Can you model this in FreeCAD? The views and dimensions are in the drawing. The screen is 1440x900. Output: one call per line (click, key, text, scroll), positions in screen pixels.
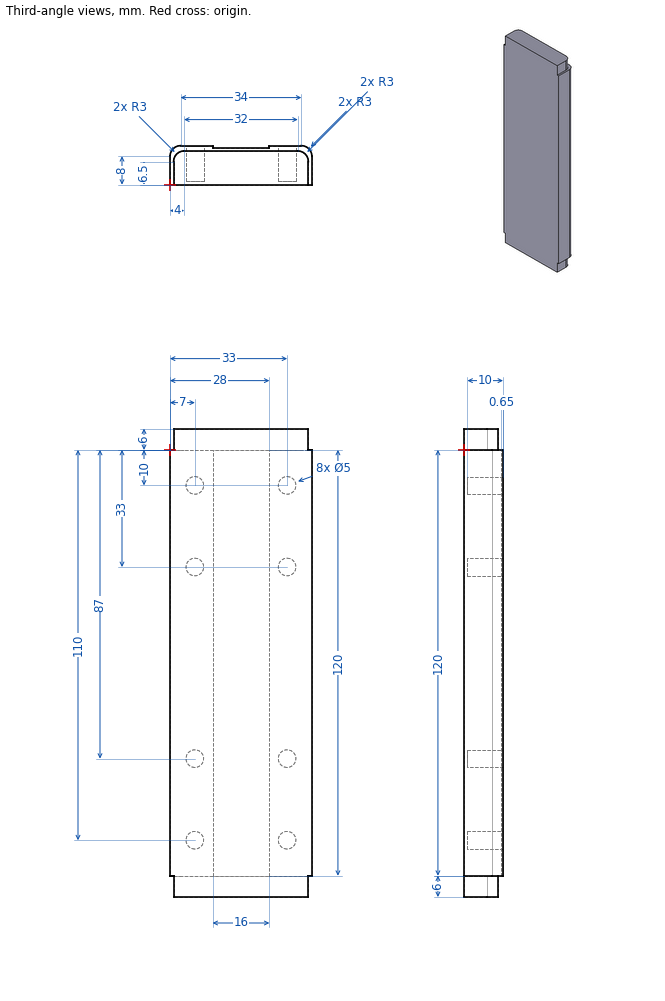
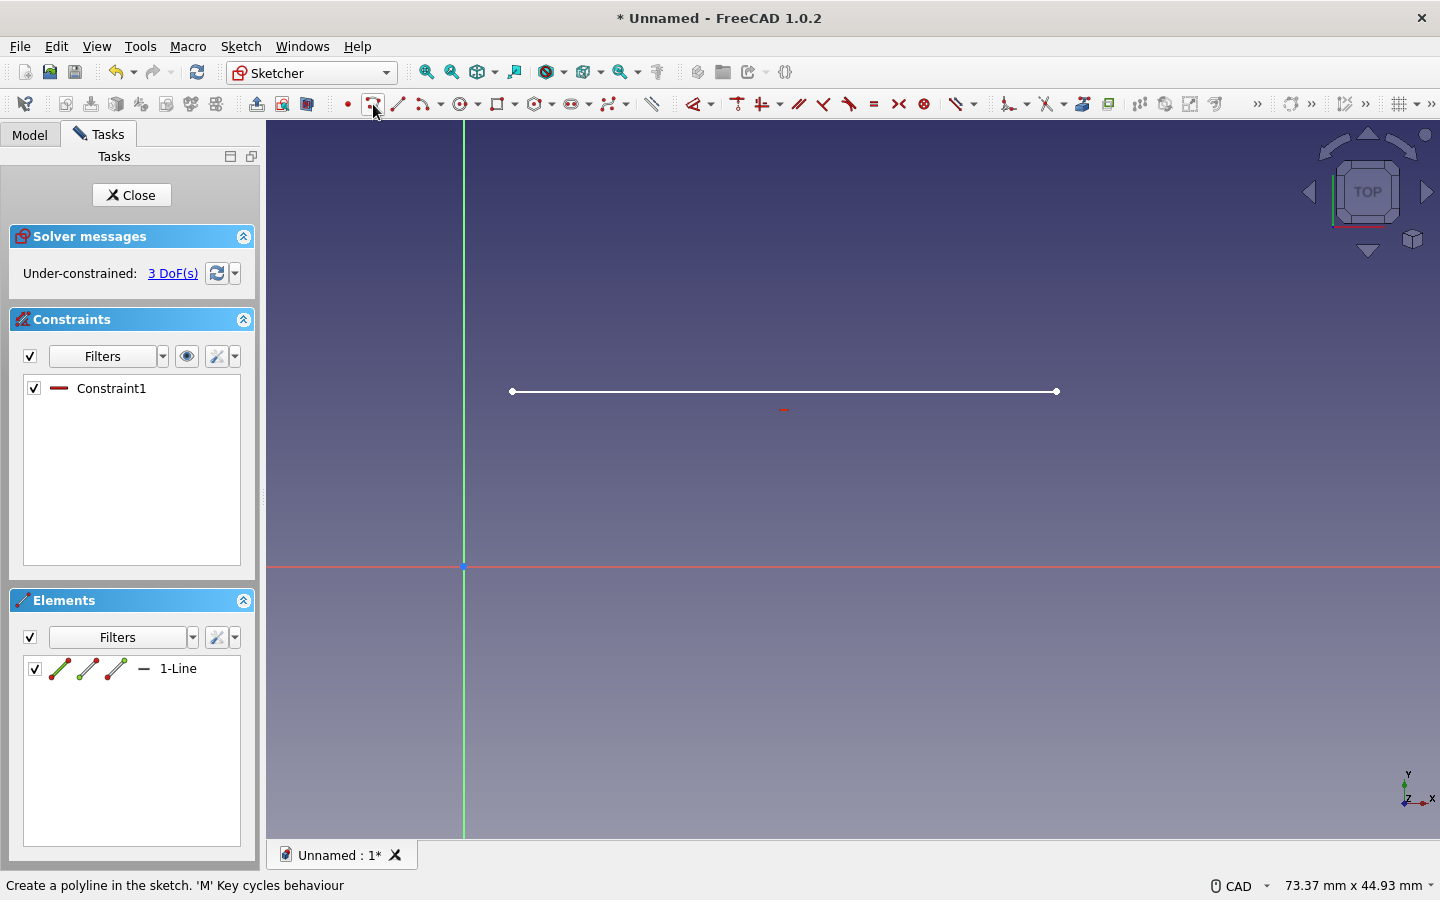
click(464, 439)
click(464, 567)
click(1104, 558)
click(1104, 439)
right_click(1104, 439)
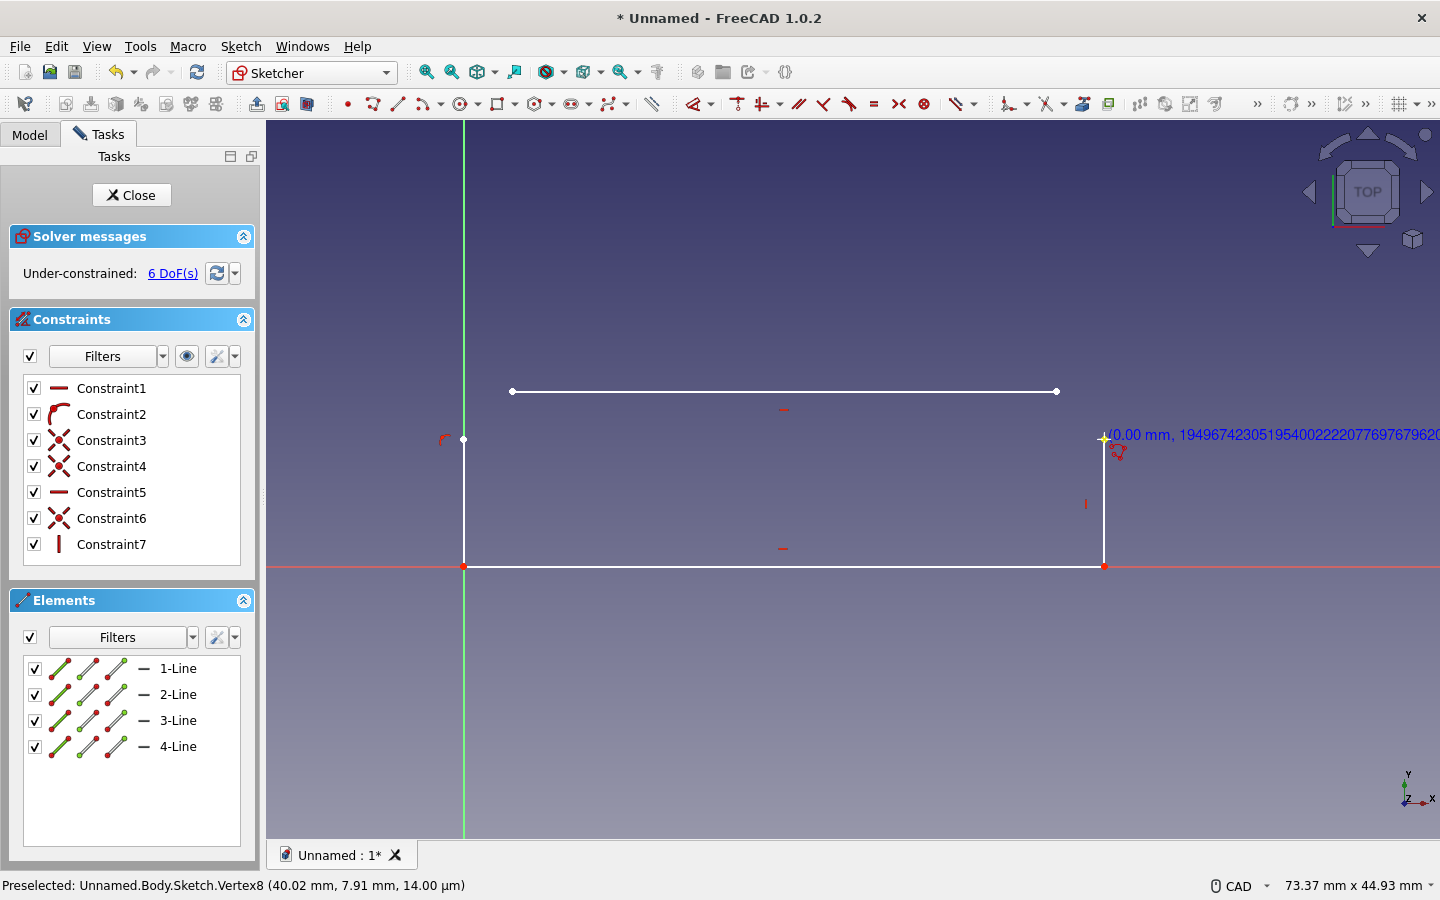
click(440, 104)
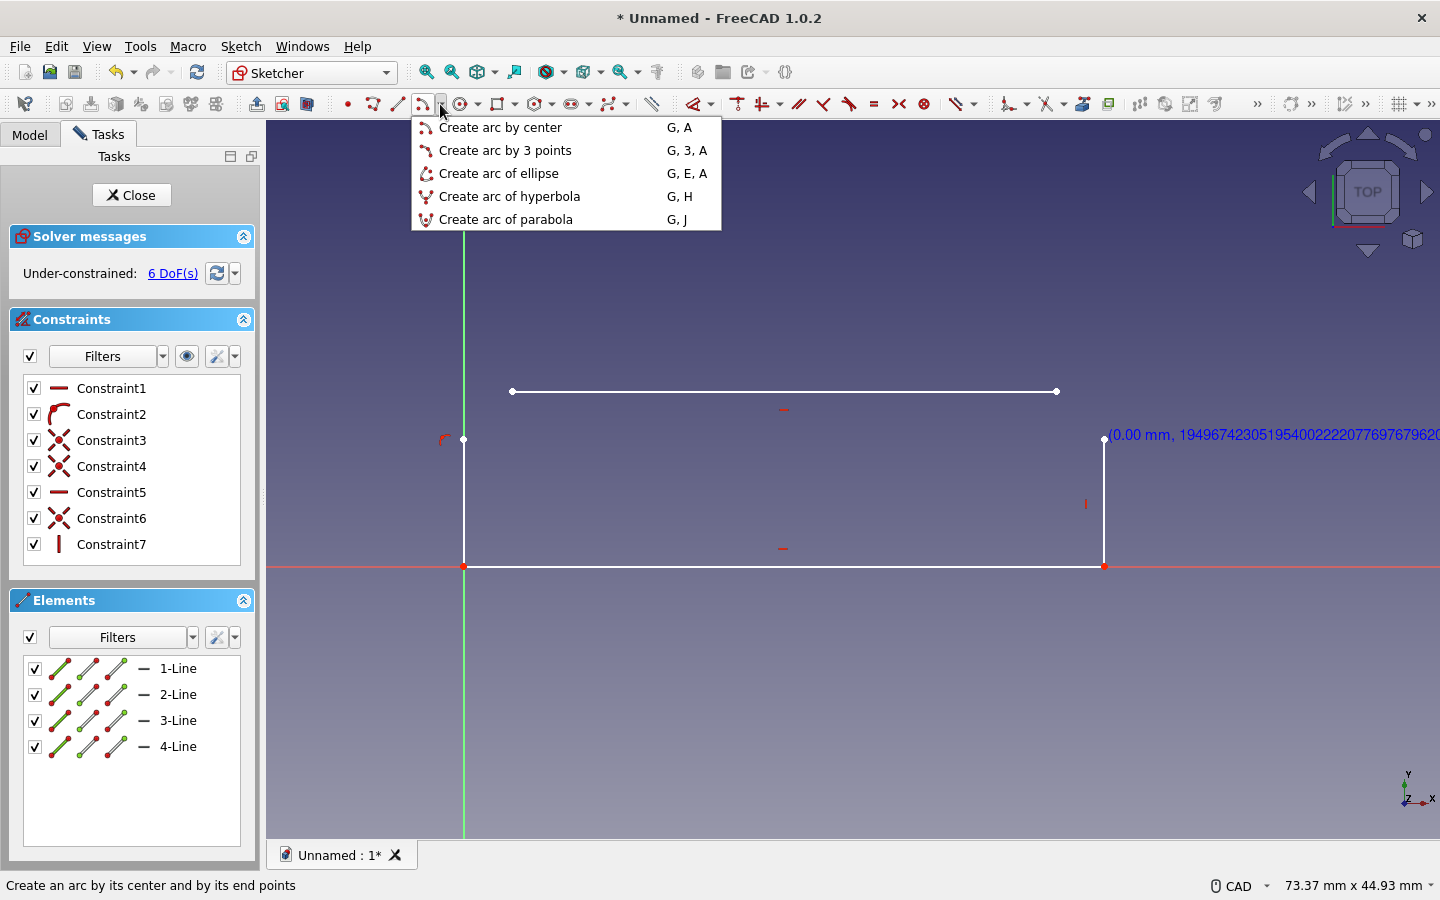
click(566, 150)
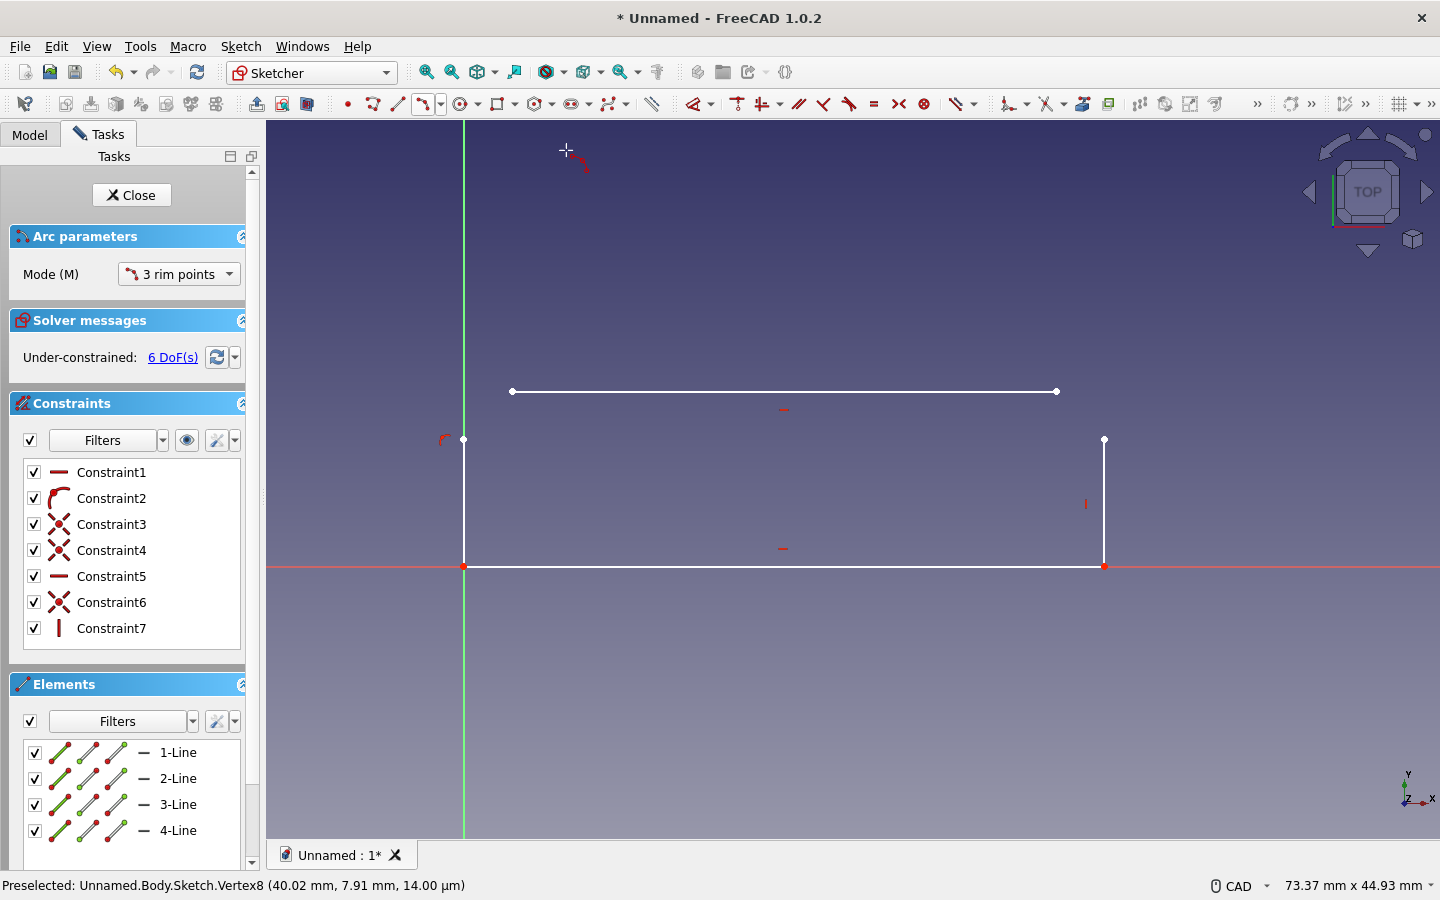
click(512, 392)
click(464, 440)
click(478, 405)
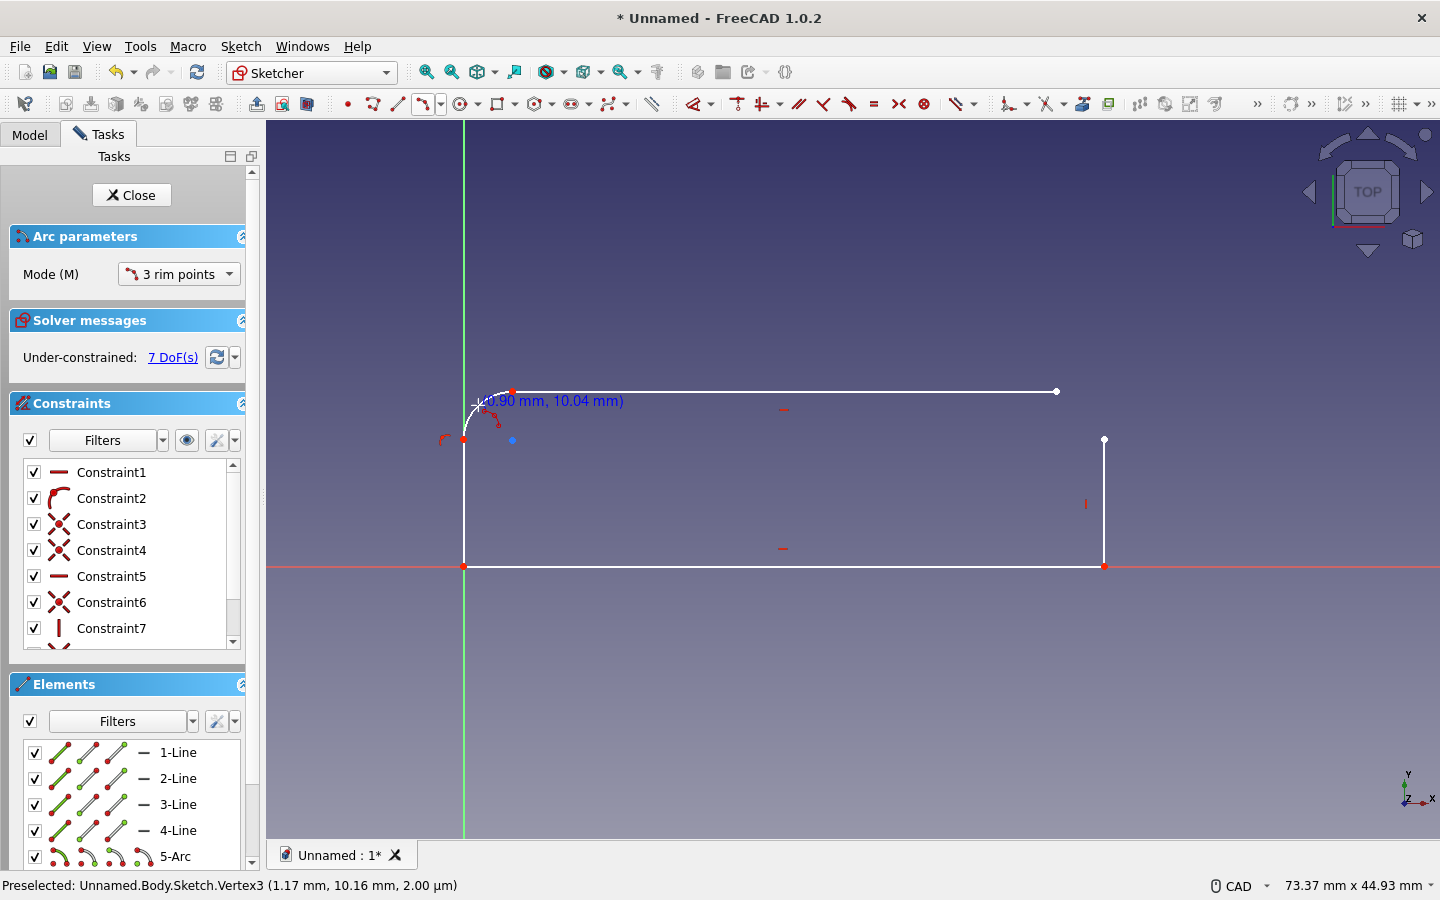
click(1104, 440)
click(1056, 392)
click(1090, 405)
key(Escape)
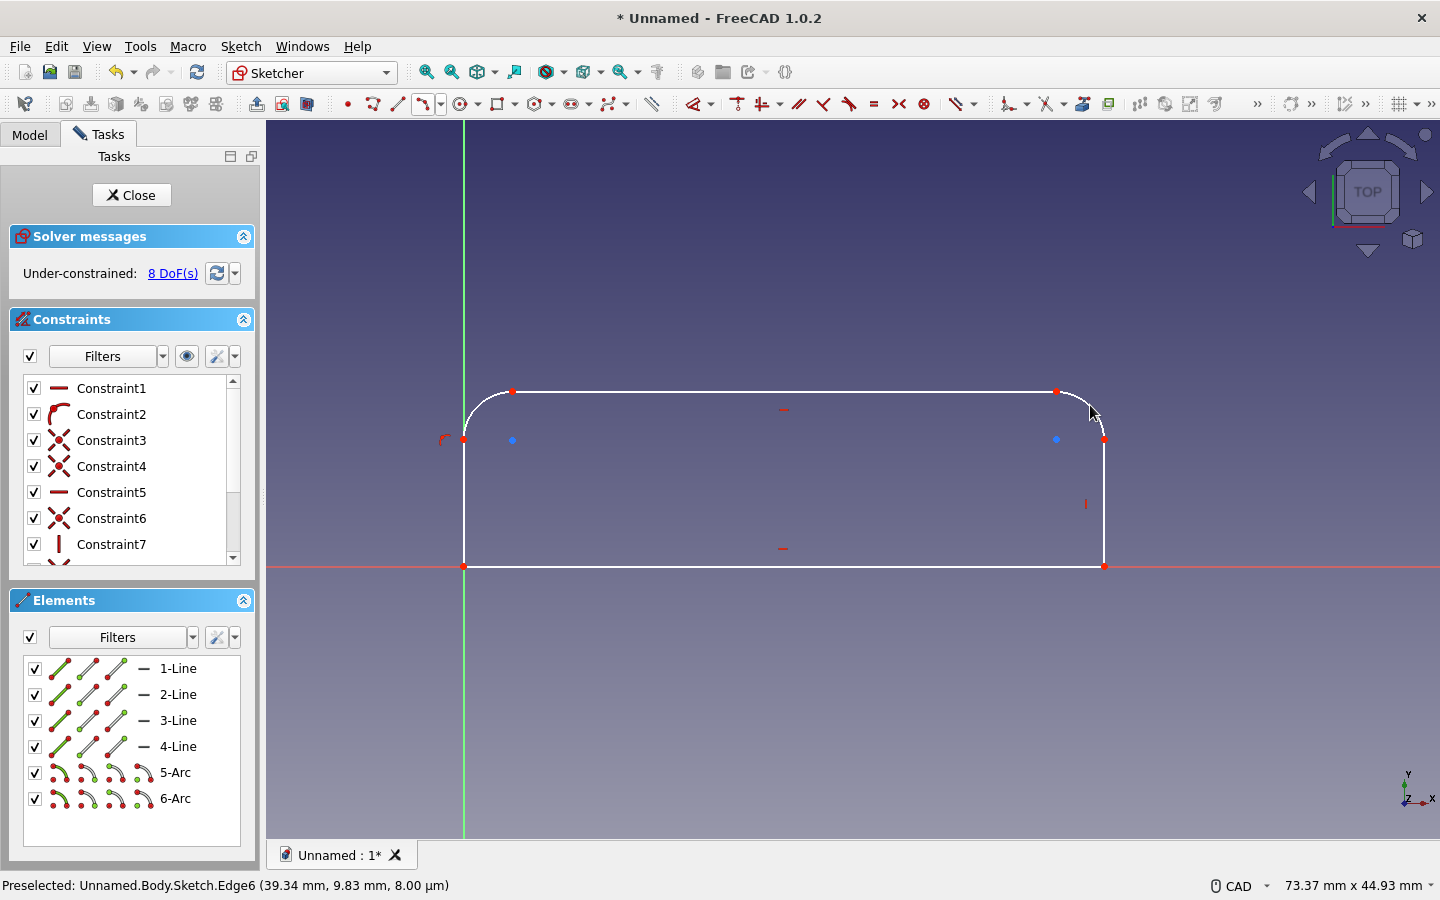
click(893, 392)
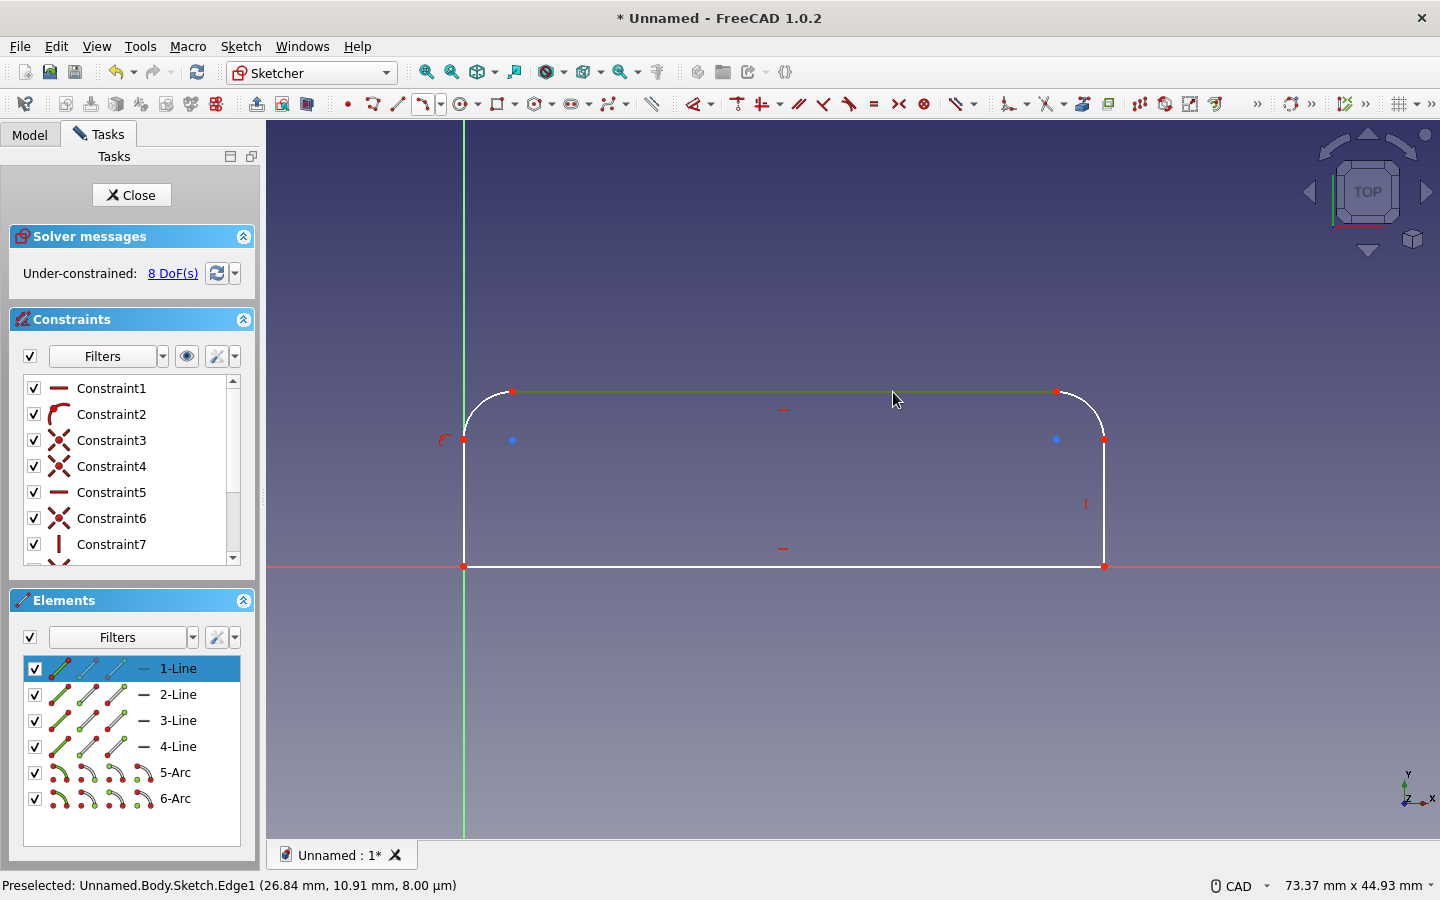
click(490, 397)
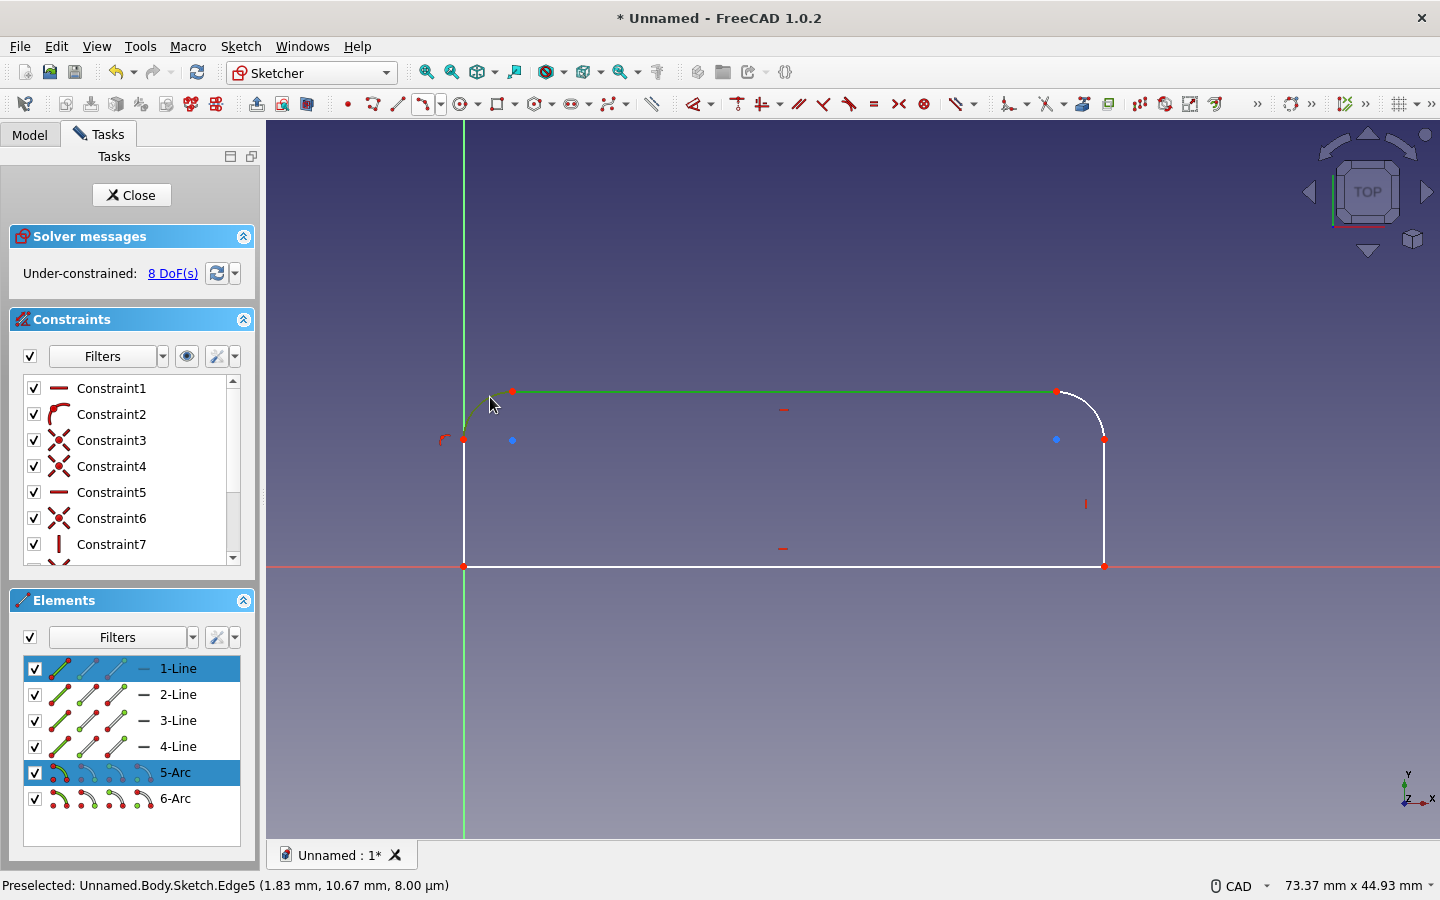
key(t)